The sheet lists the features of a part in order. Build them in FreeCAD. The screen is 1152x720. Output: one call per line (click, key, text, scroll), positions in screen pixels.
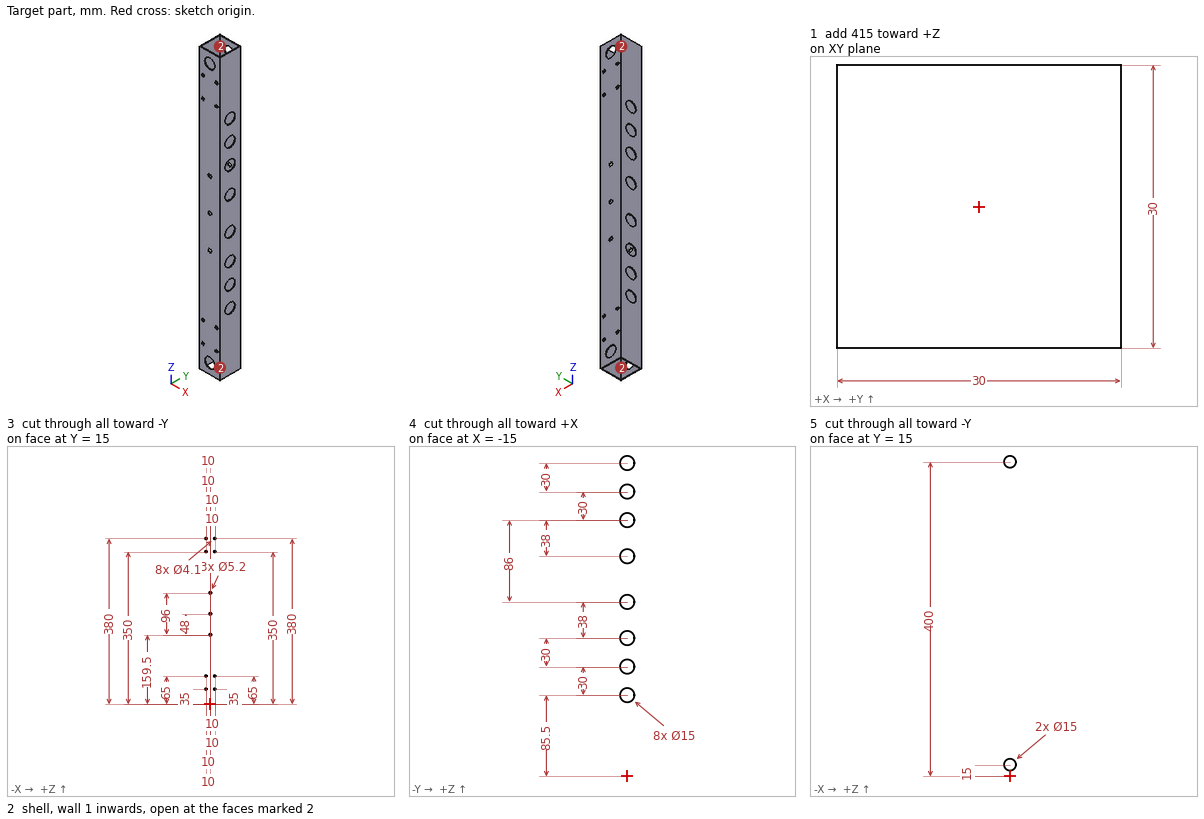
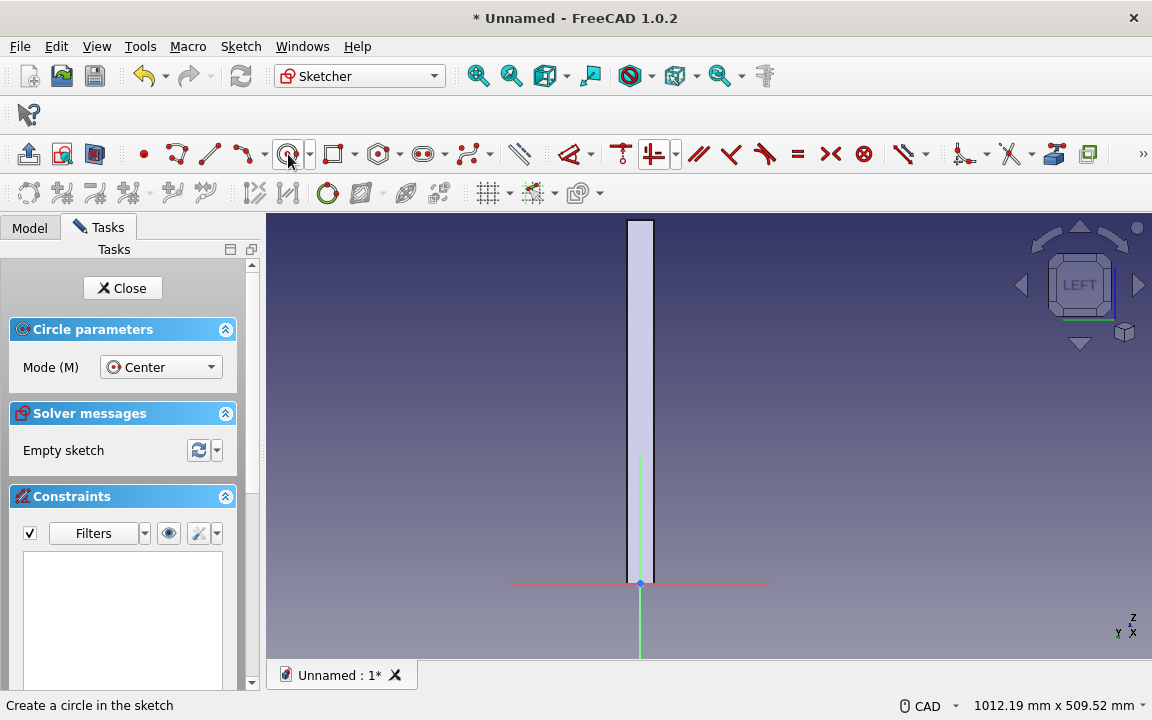
scroll(640, 509, up, 7)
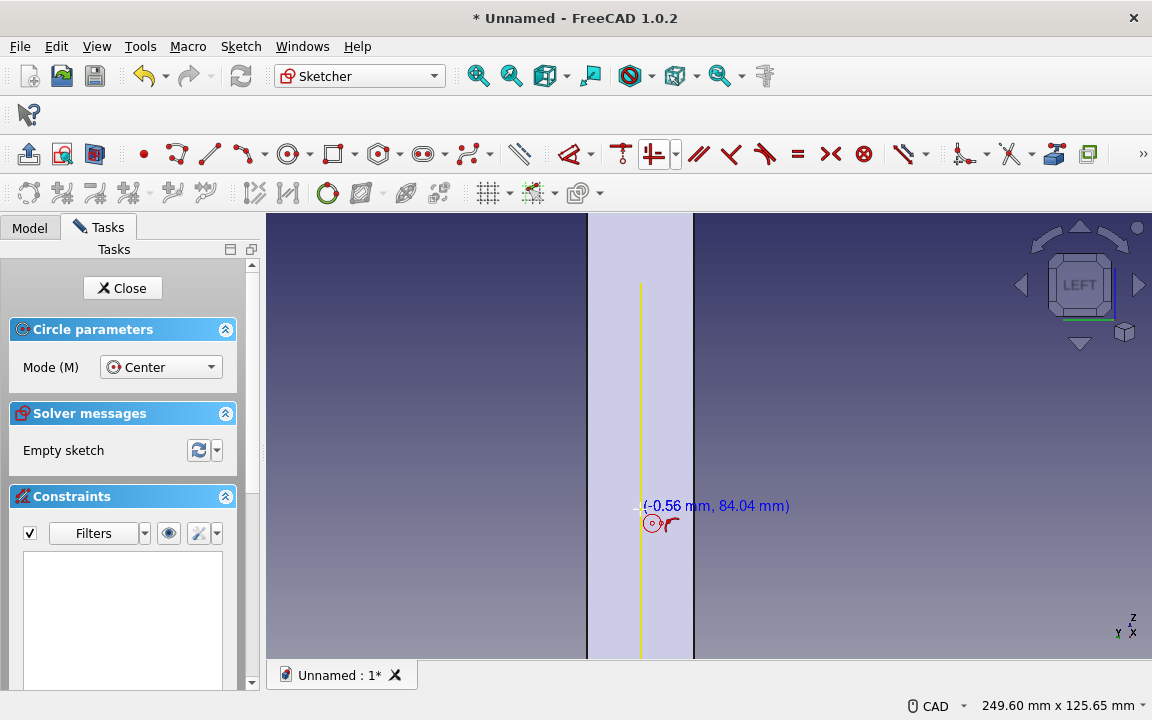
scroll(640, 510, down, 7)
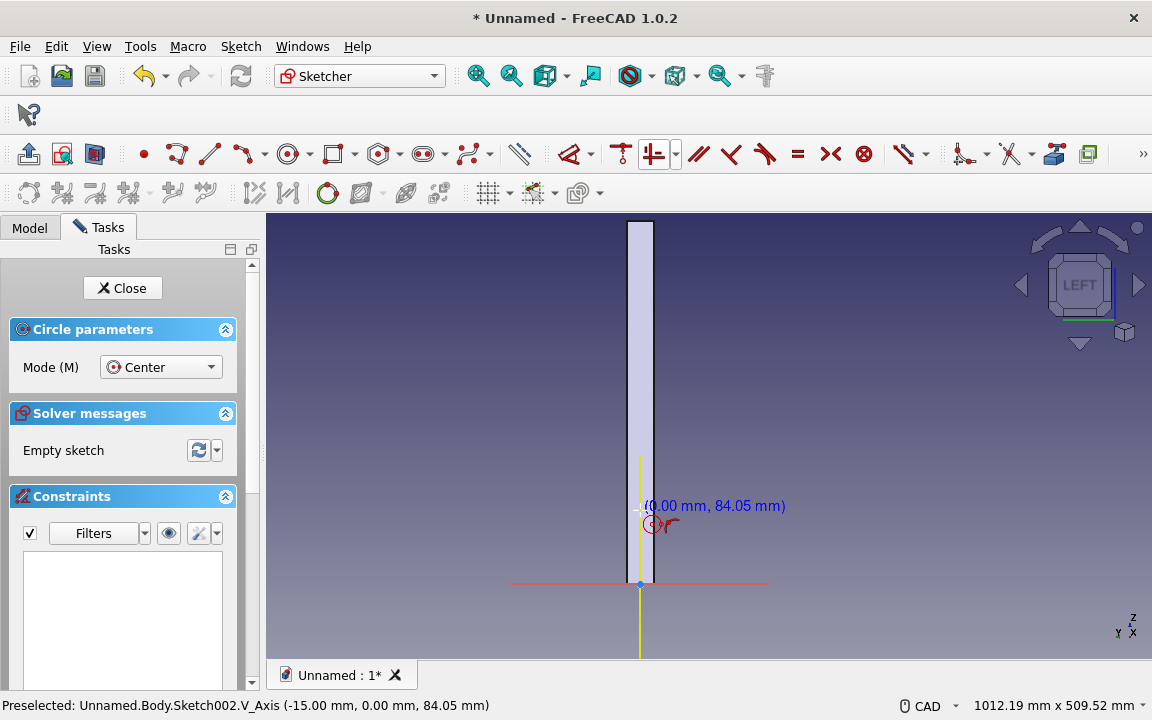
click(640, 509)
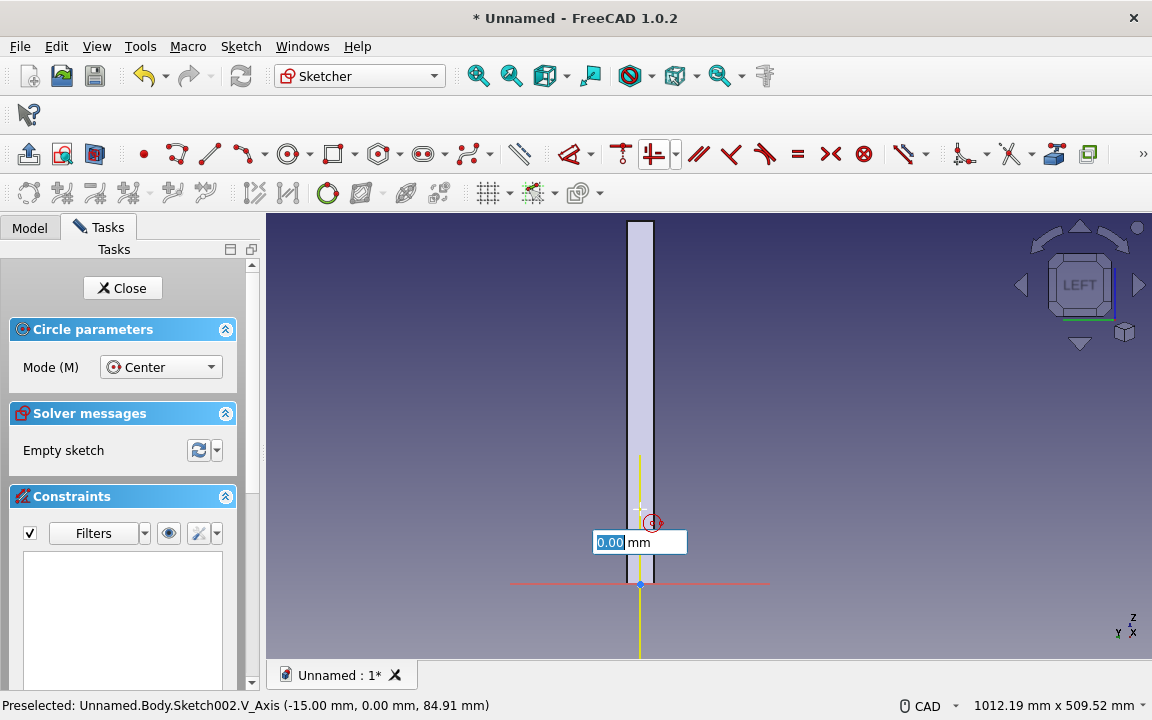
scroll(647, 507, up, 5)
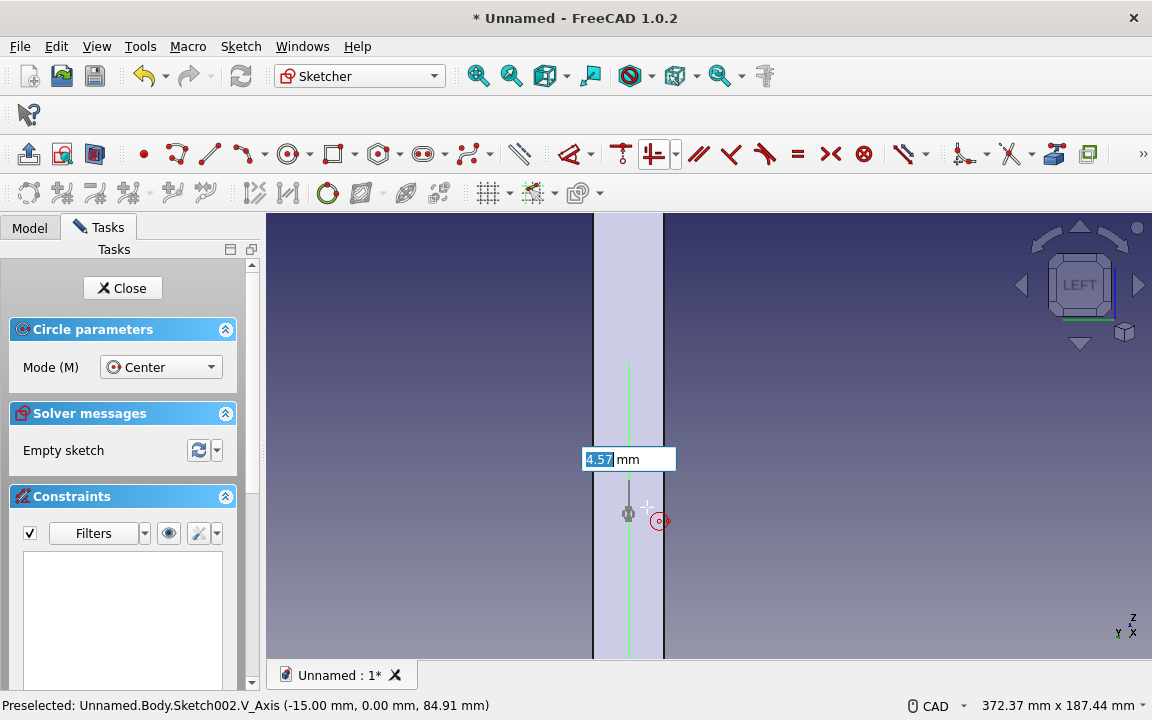
click(645, 507)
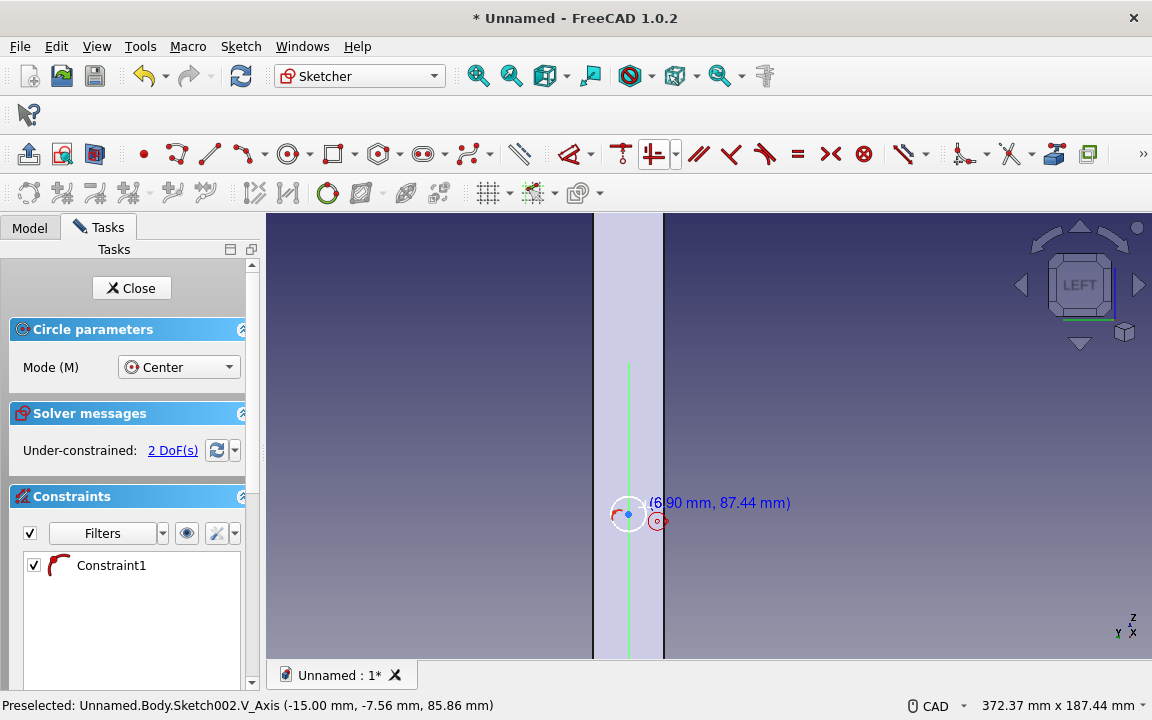
scroll(629, 441, up, 2)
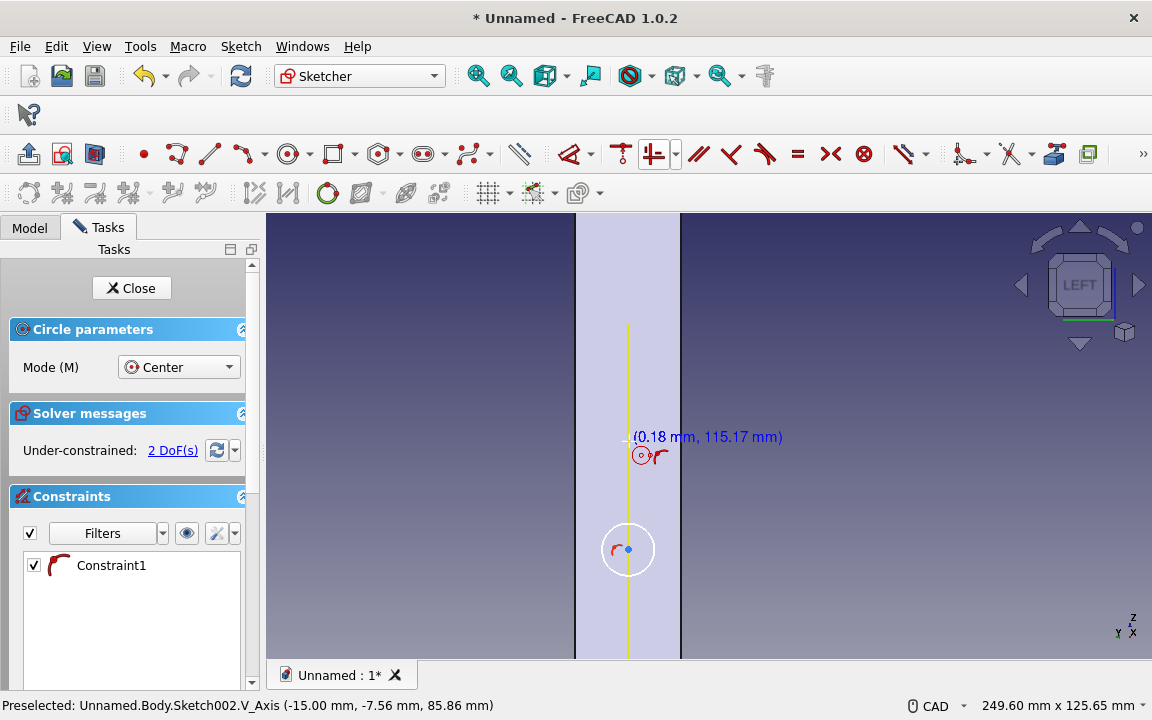
scroll(645, 496, down, 7)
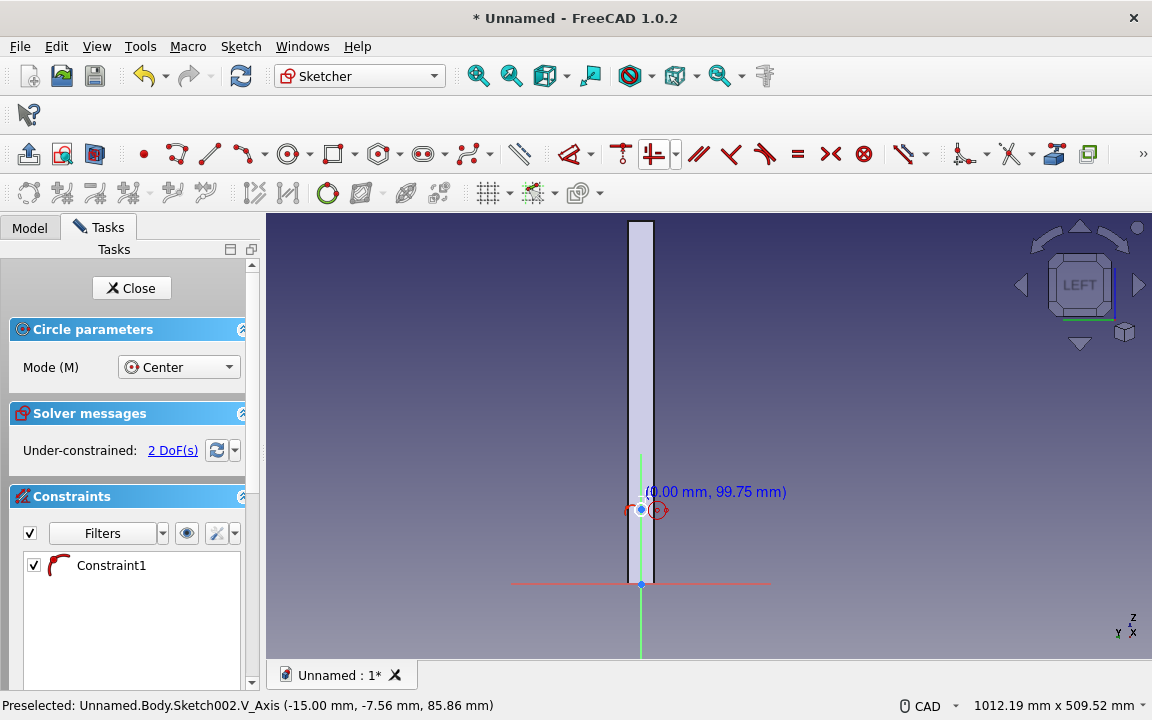
click(641, 483)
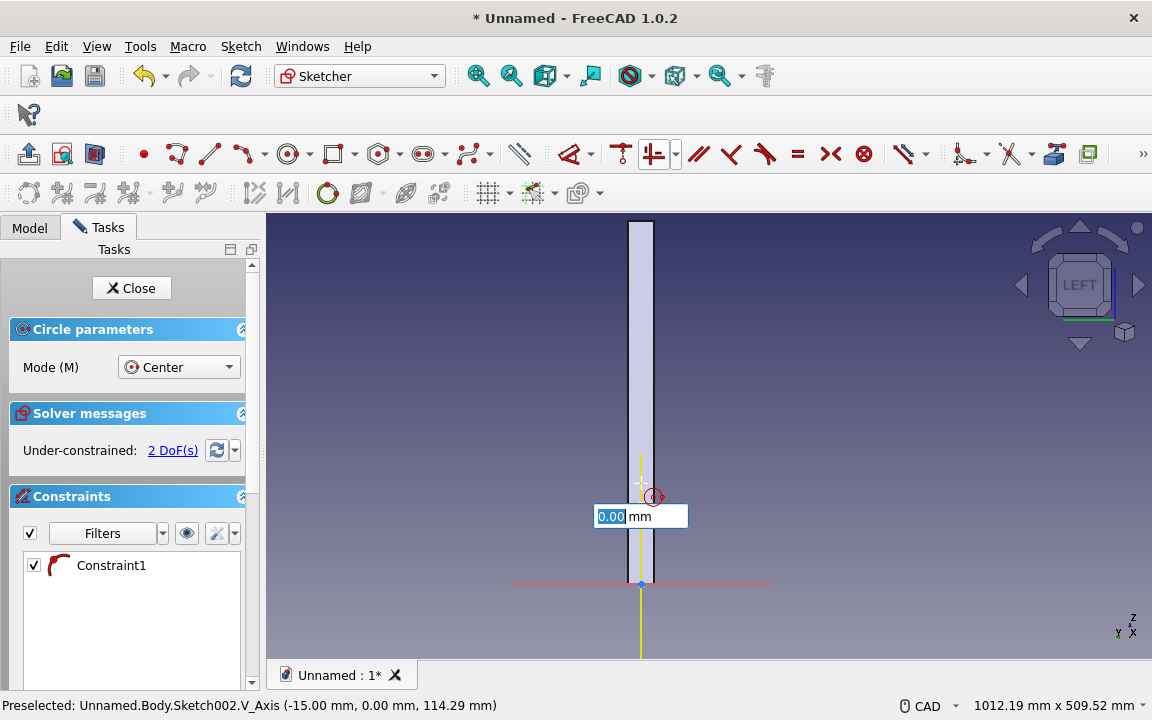
scroll(647, 481, up, 5)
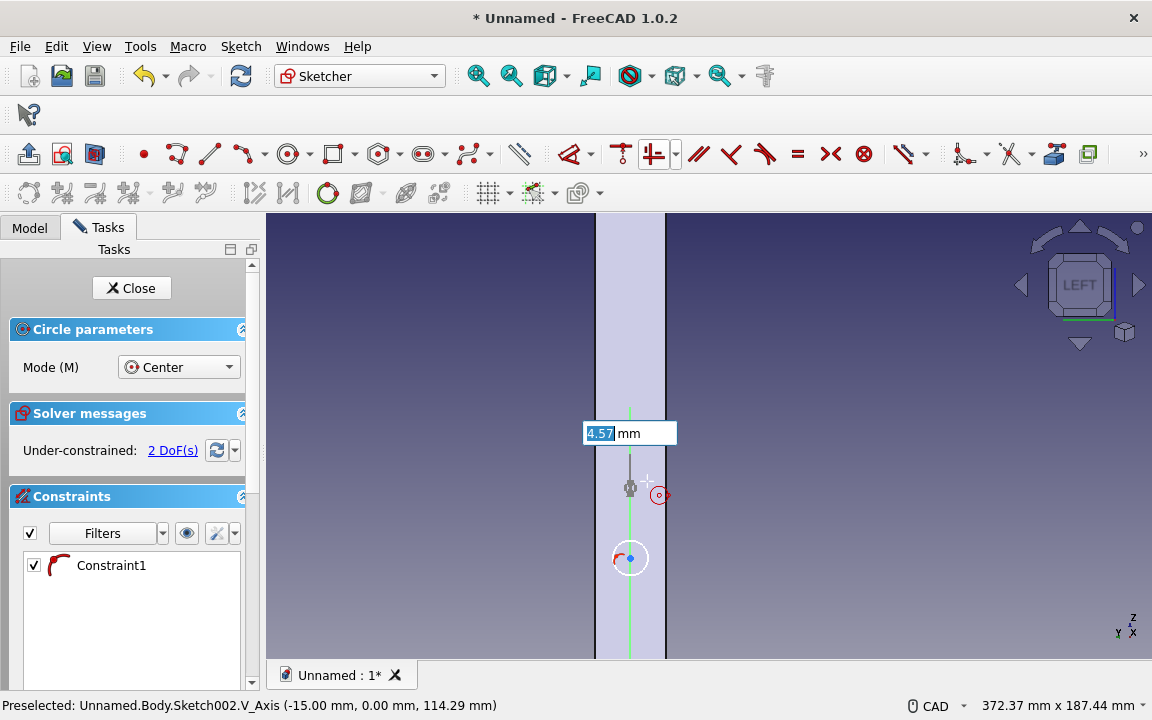
click(647, 479)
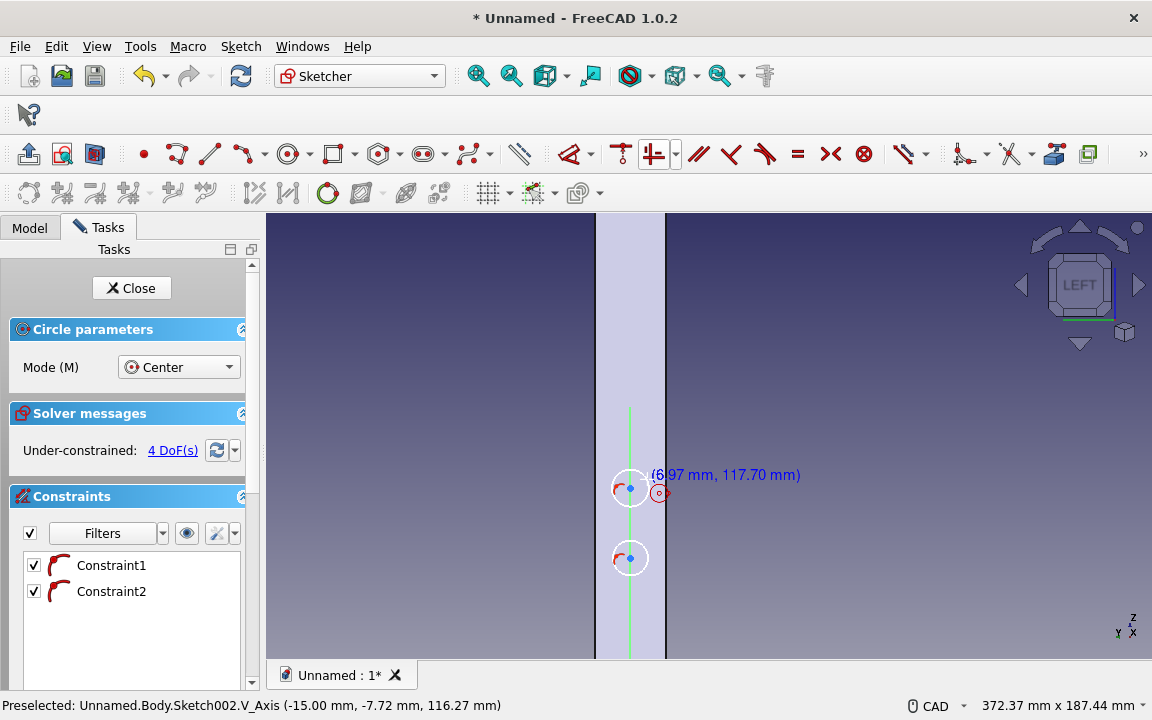
scroll(630, 414, up, 2)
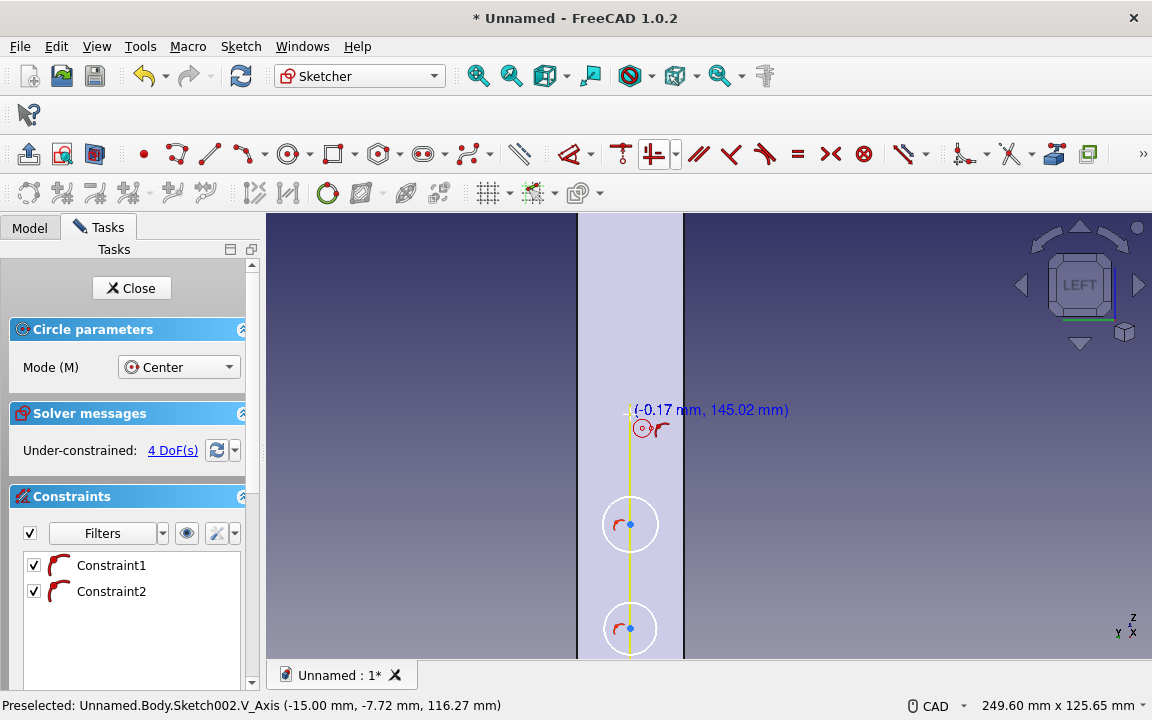
scroll(644, 470, down, 7)